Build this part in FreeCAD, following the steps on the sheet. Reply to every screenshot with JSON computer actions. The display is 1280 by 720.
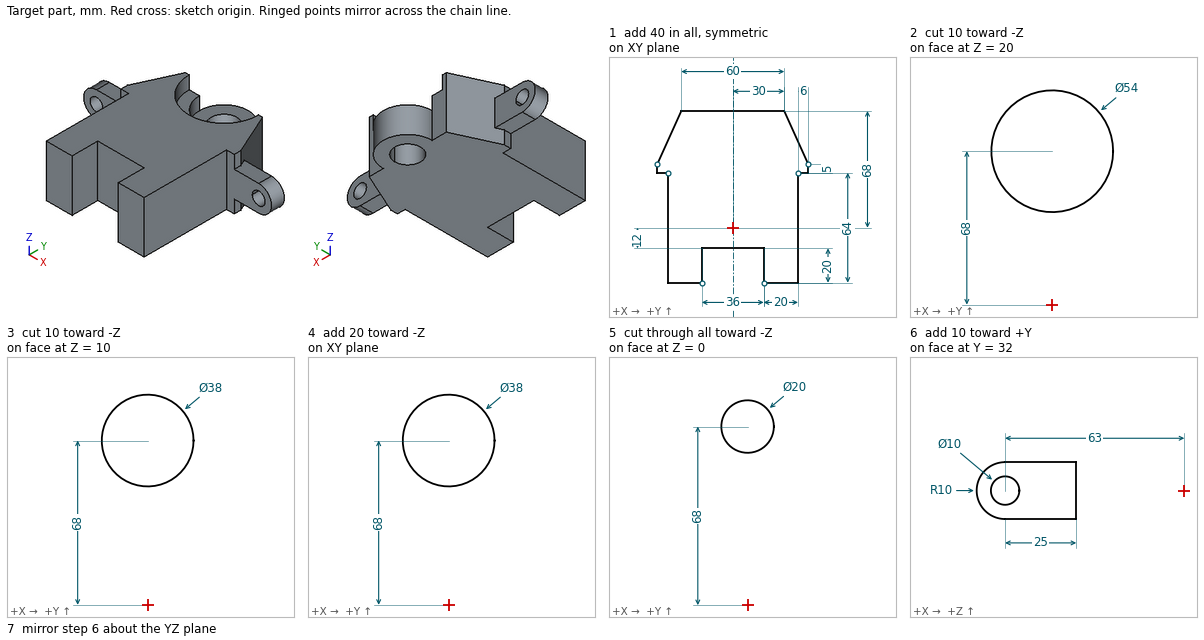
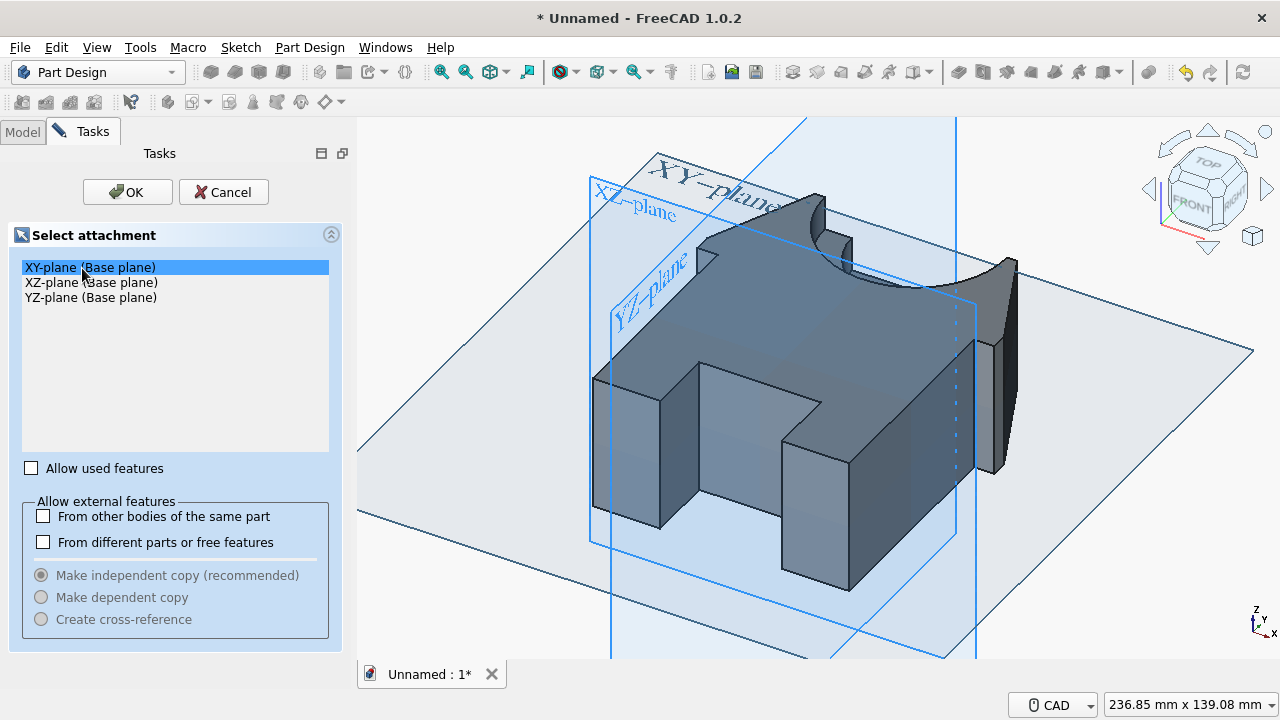
{"action": "left_click", "coordinate": [128, 192]}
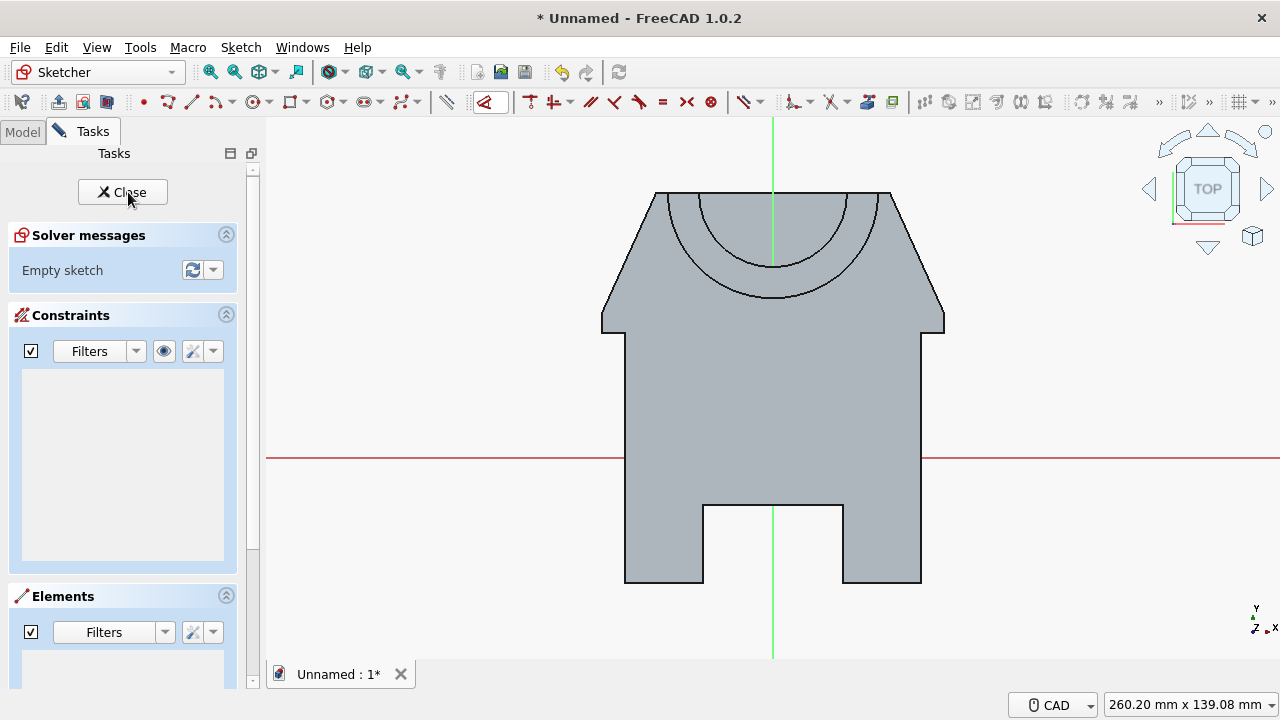
{"action": "left_click", "coordinate": [108, 102]}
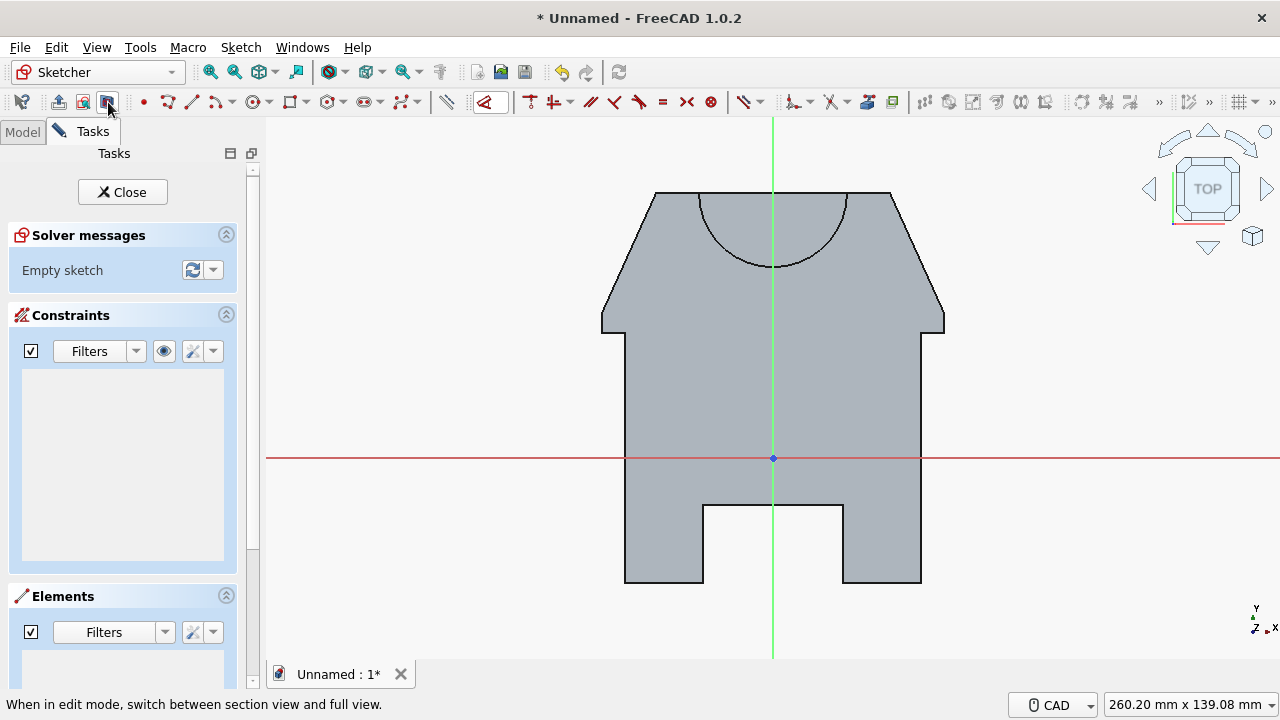
{"action": "scroll", "coordinate": [395, 631], "scroll_direction": "down", "scroll_amount": 1}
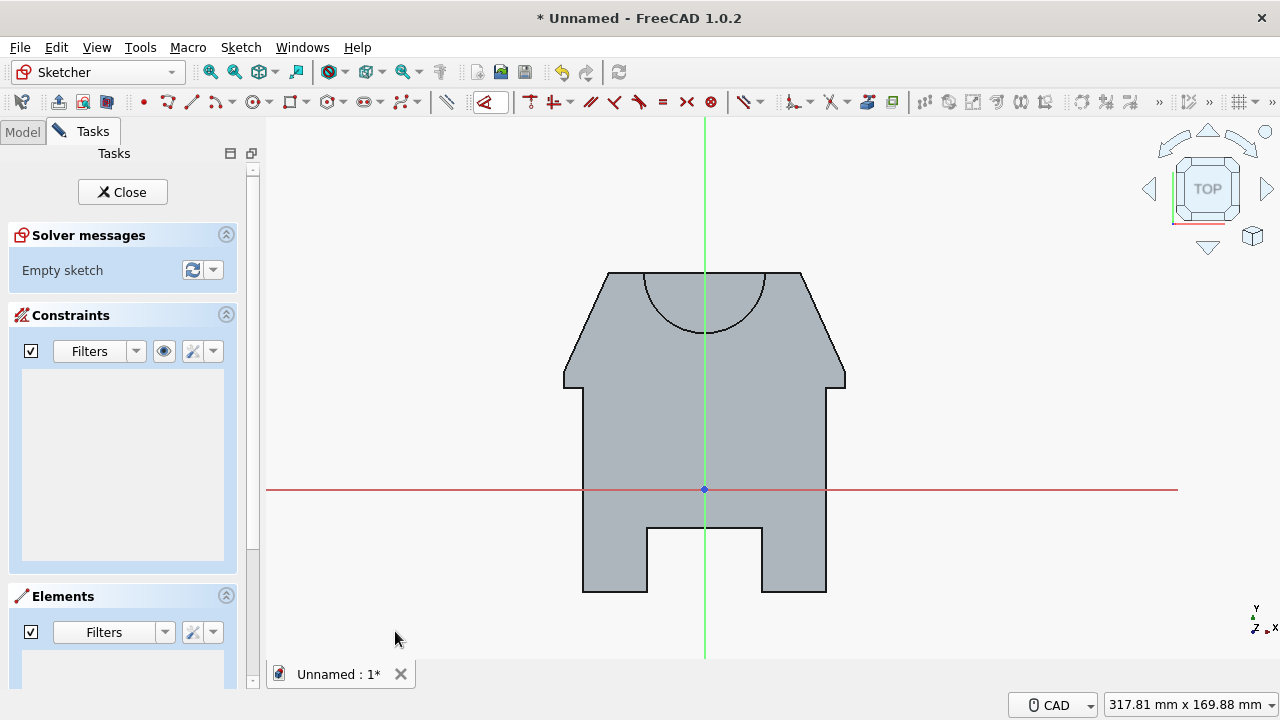
{"action": "left_click", "coordinate": [254, 102]}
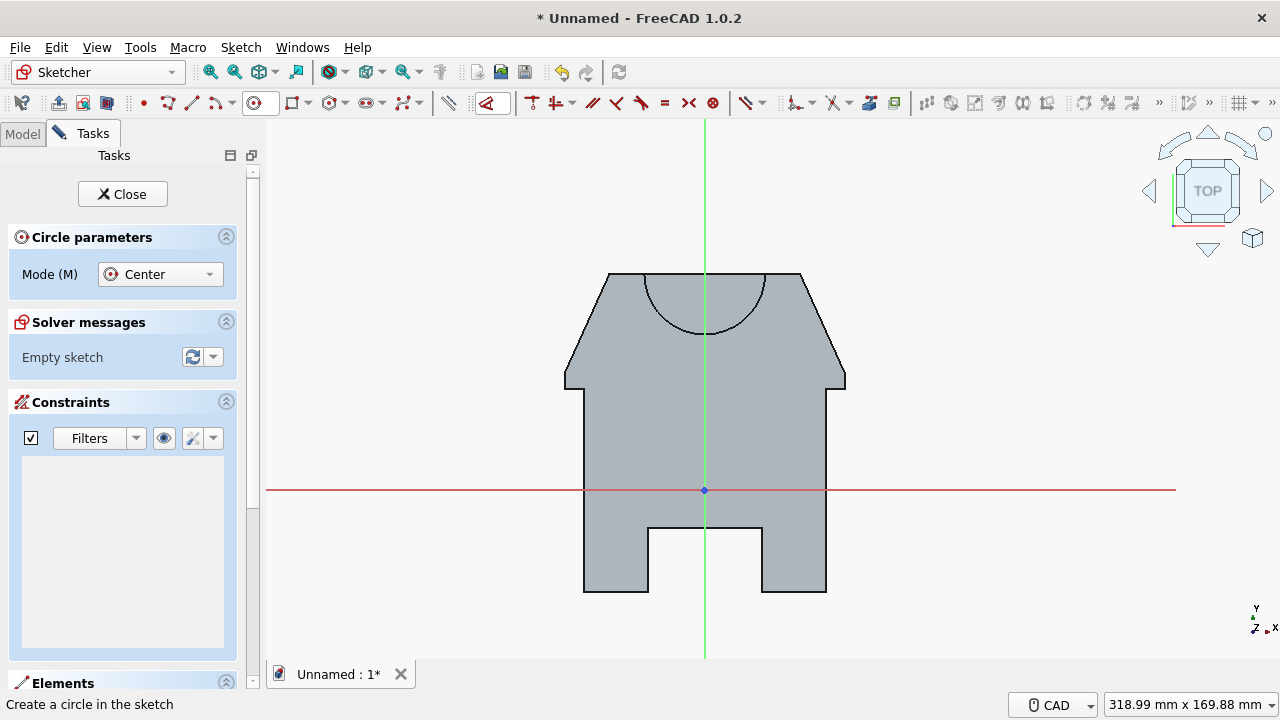
{"action": "left_click", "coordinate": [705, 274]}
{"action": "left_click", "coordinate": [747, 231]}
{"action": "key", "text": "Escape"}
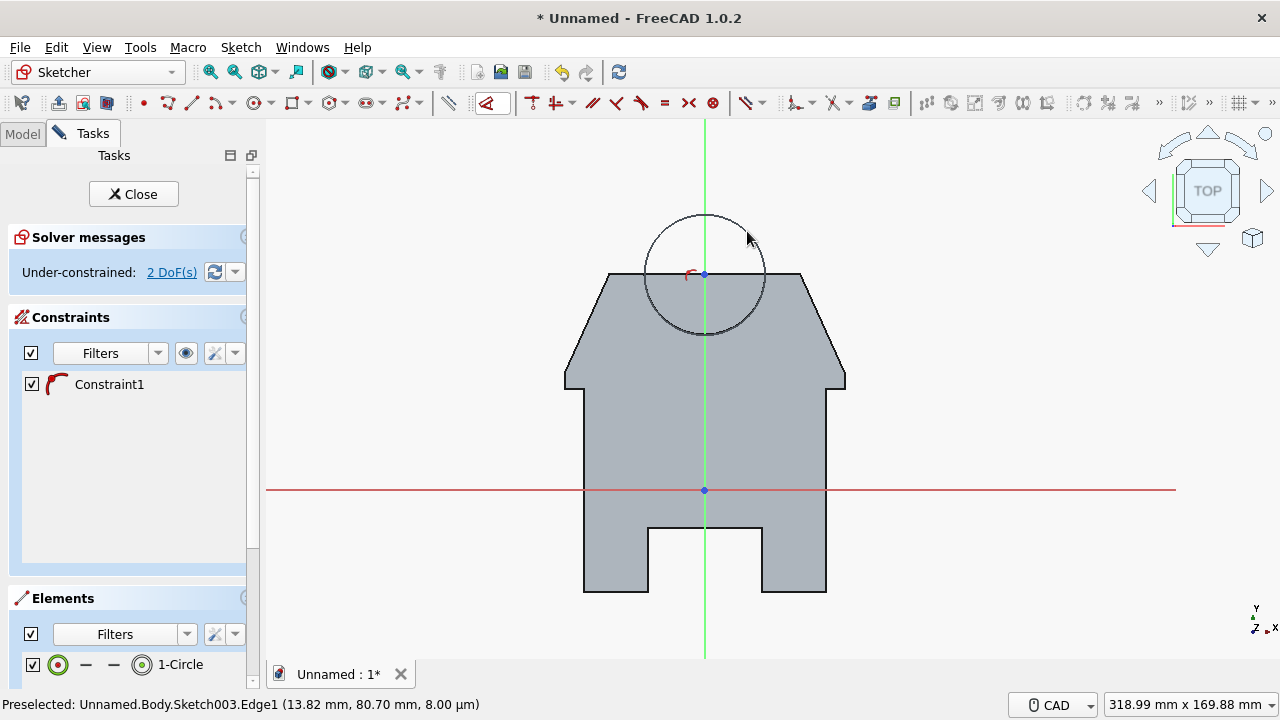
{"action": "left_click", "coordinate": [747, 232]}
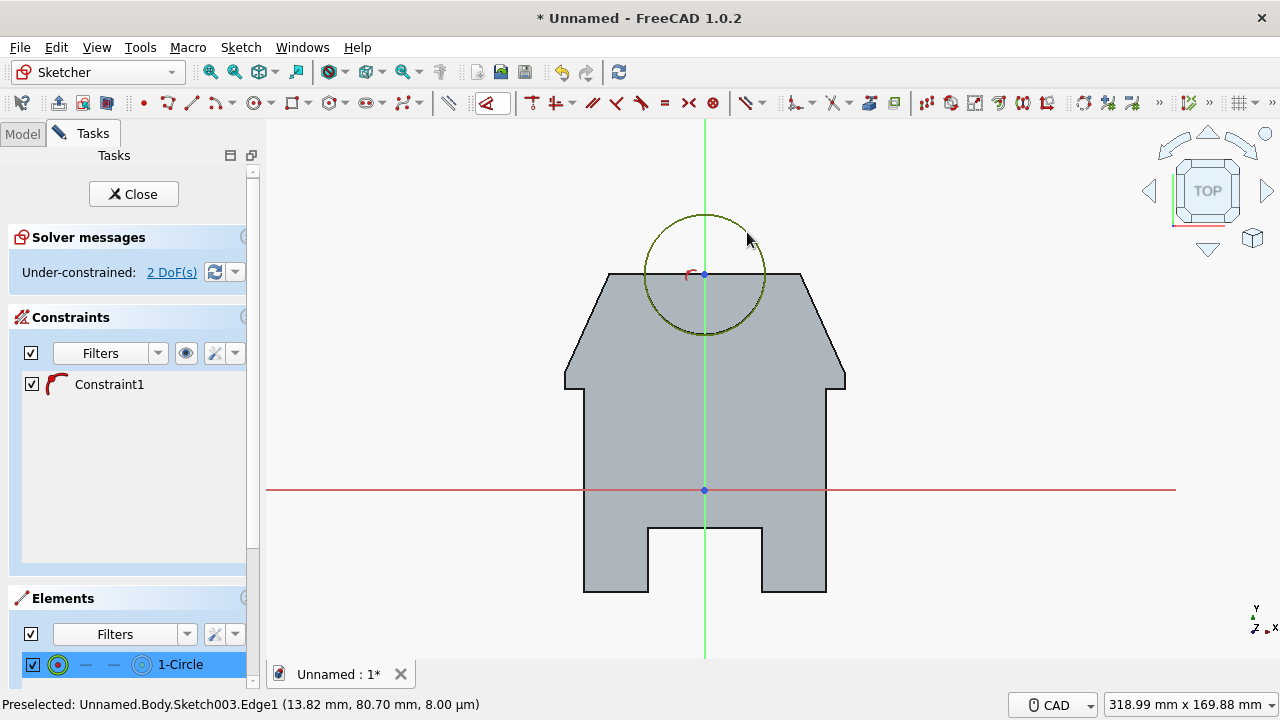
{"action": "key", "text": "k o"}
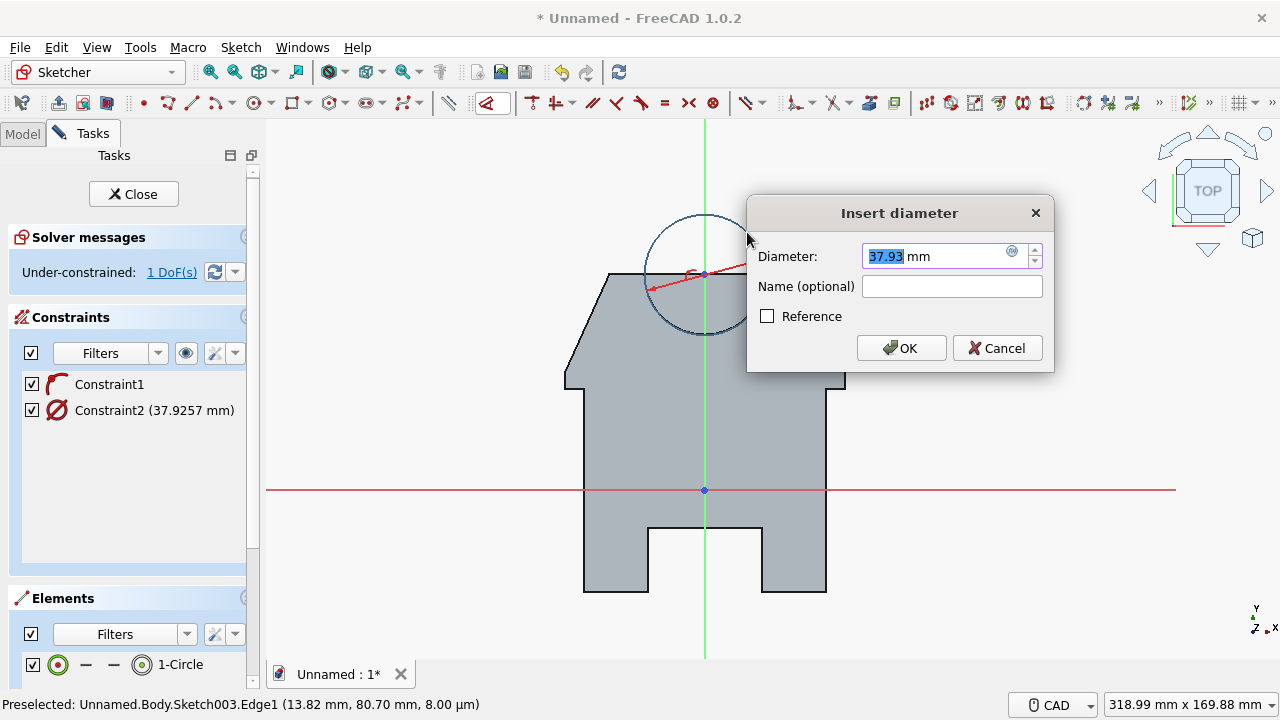
{"action": "type", "text": "38"}
{"action": "key", "text": "Return"}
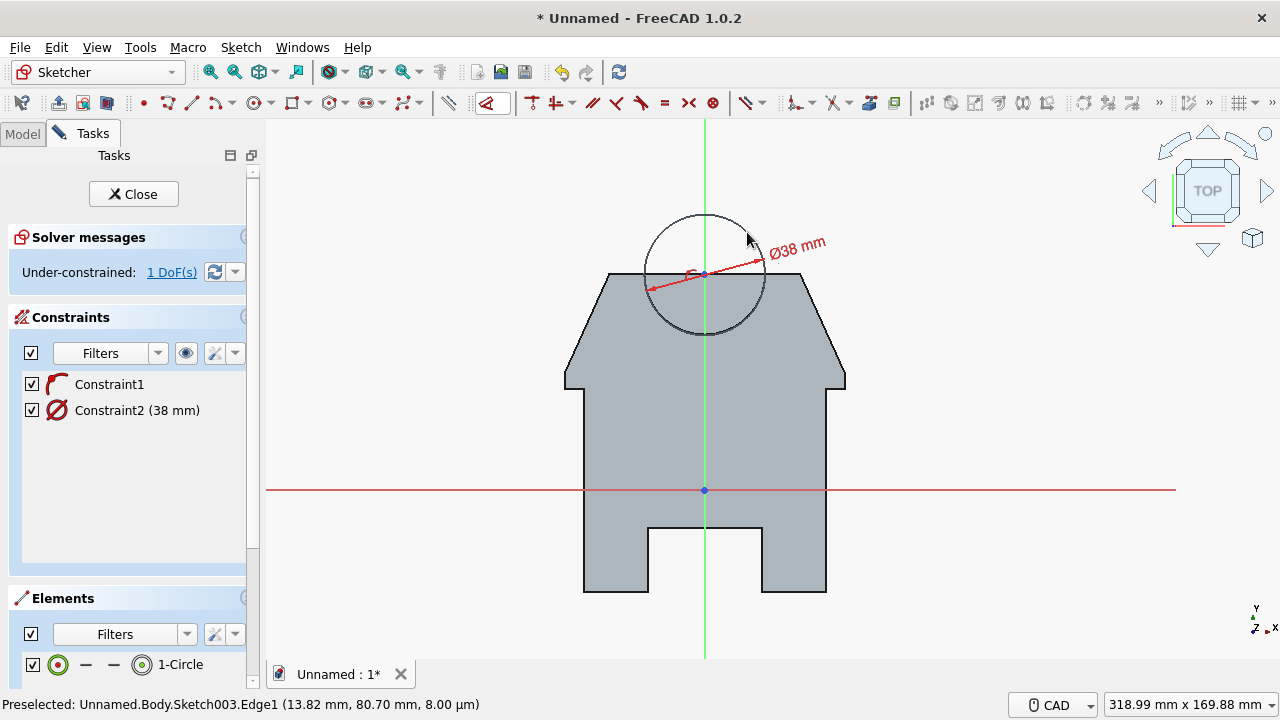
{"action": "left_click", "coordinate": [705, 275]}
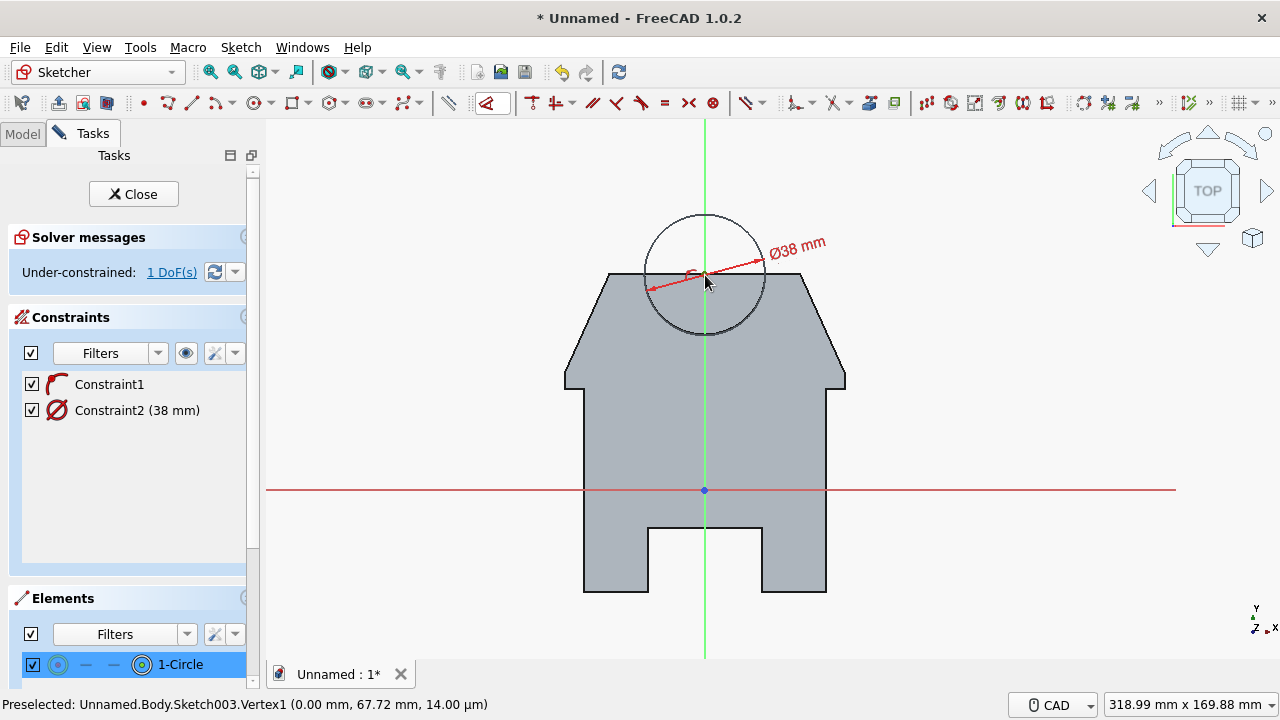
{"action": "left_click", "coordinate": [504, 104]}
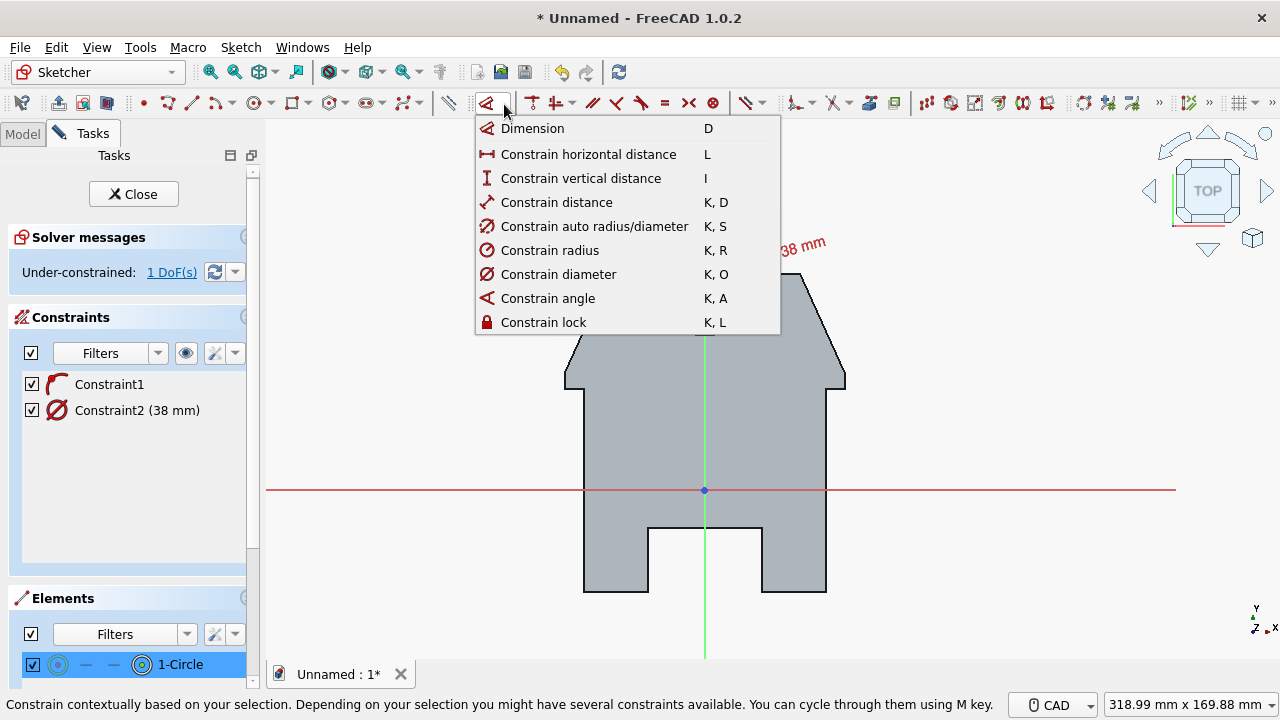
{"action": "left_click", "coordinate": [628, 178]}